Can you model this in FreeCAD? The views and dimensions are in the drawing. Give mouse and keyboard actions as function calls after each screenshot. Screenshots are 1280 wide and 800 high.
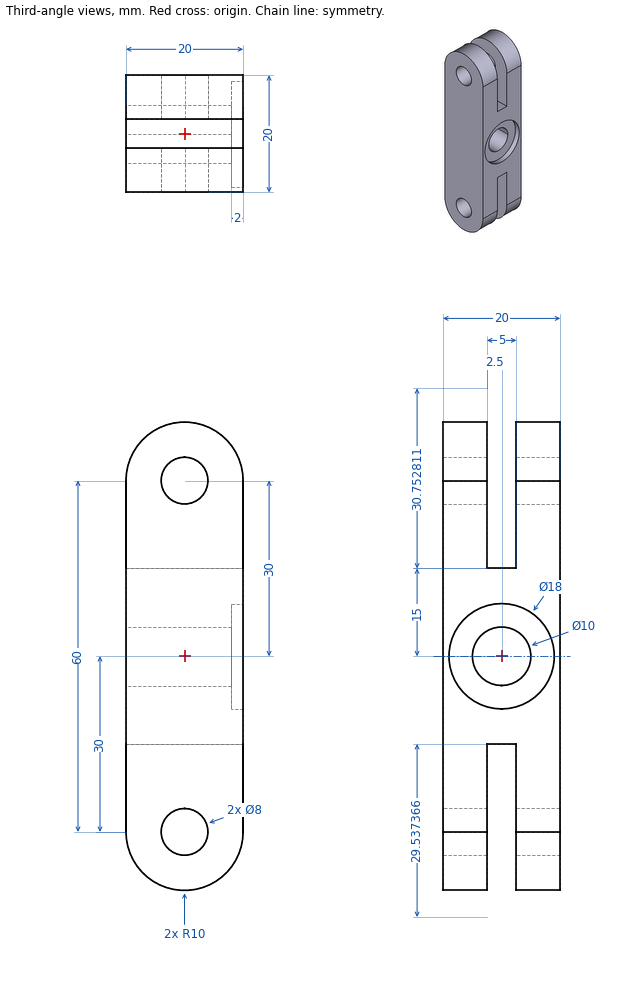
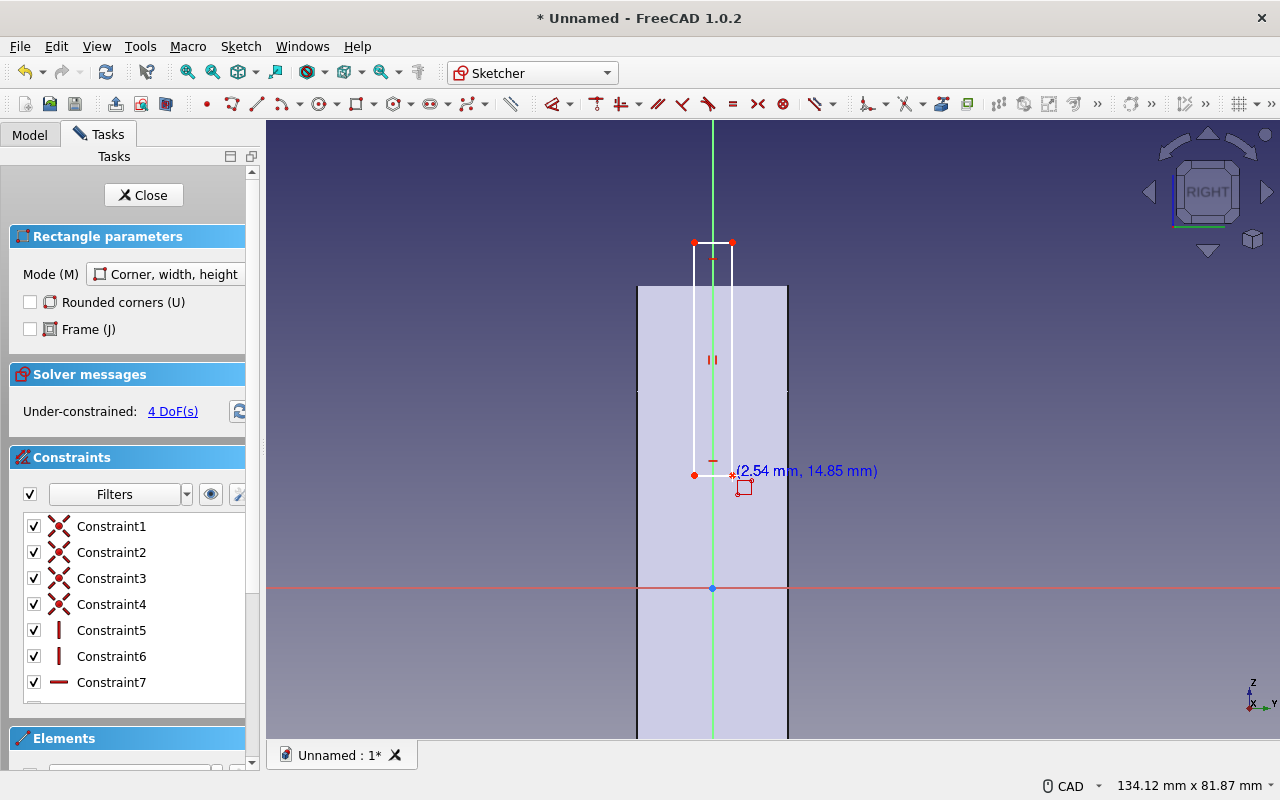
click(694, 702)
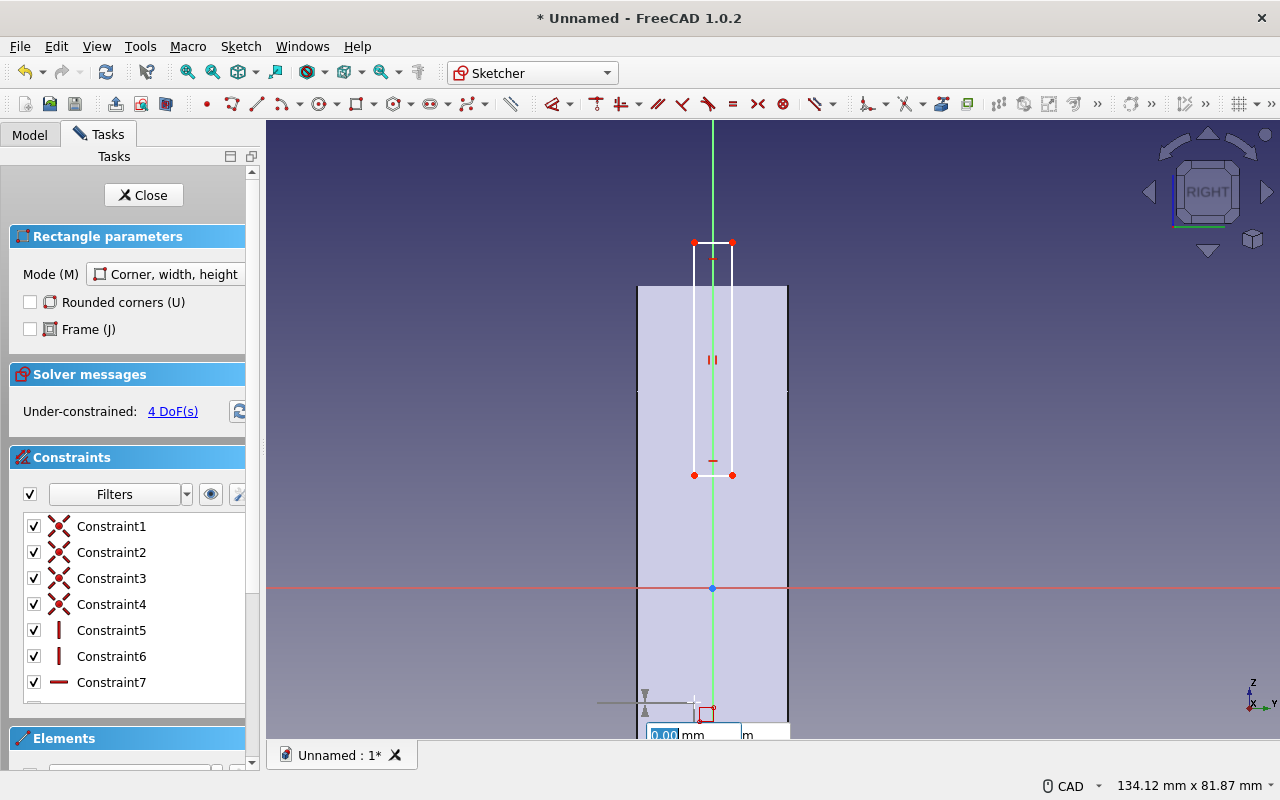
scroll(694, 242, down, 3)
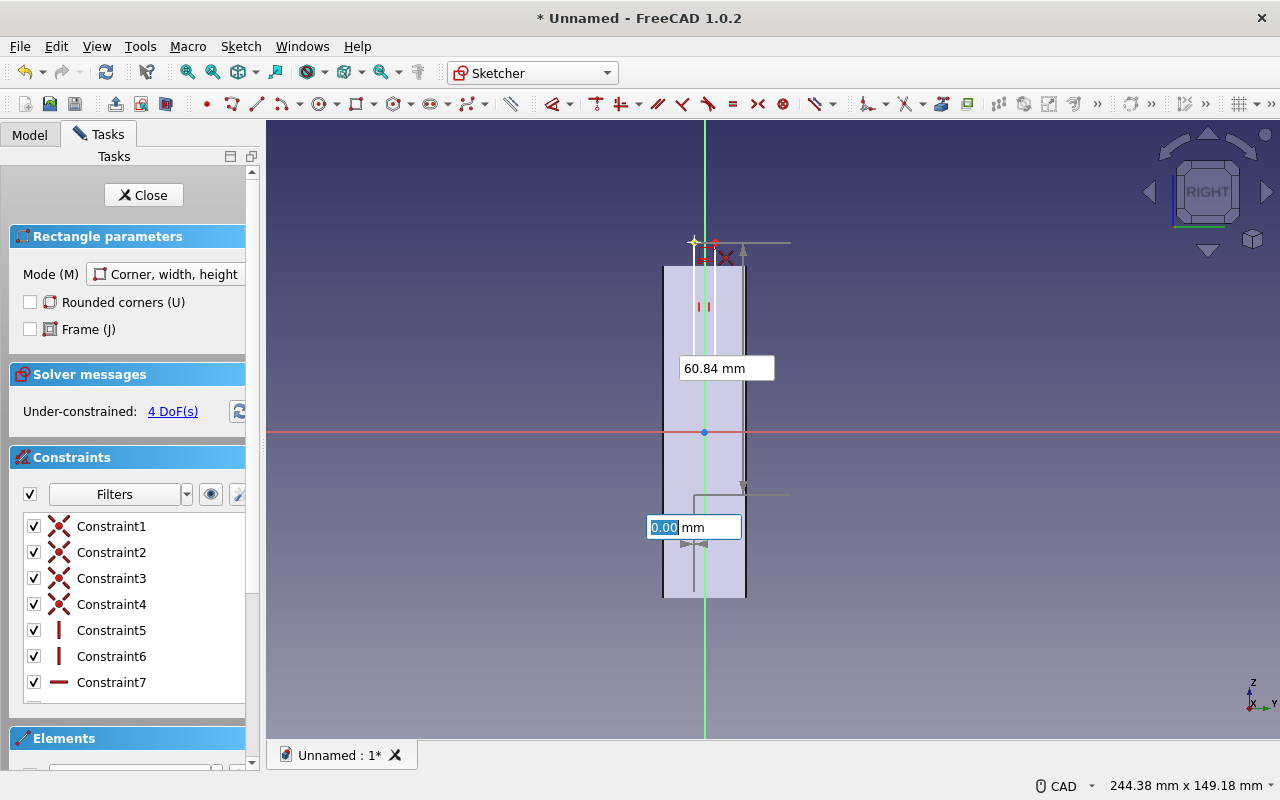
scroll(715, 617, up, 3)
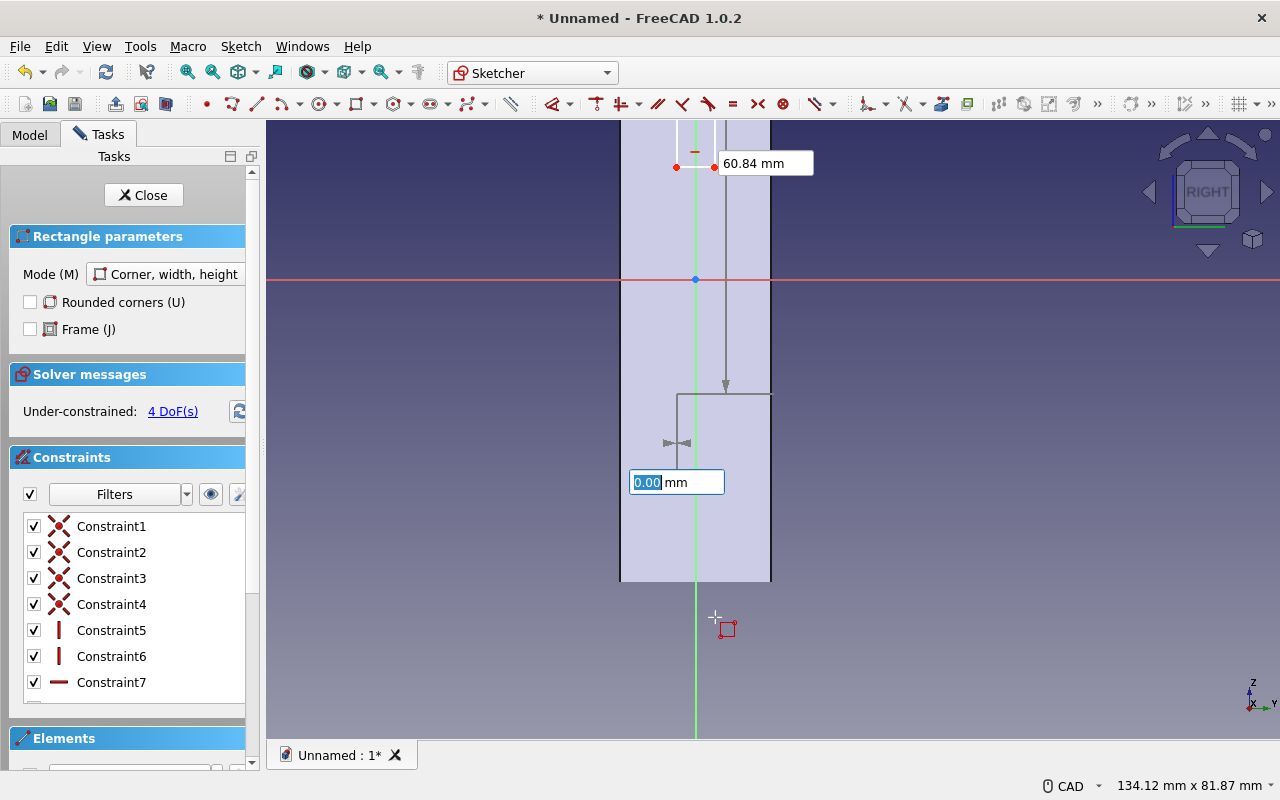
click(714, 616)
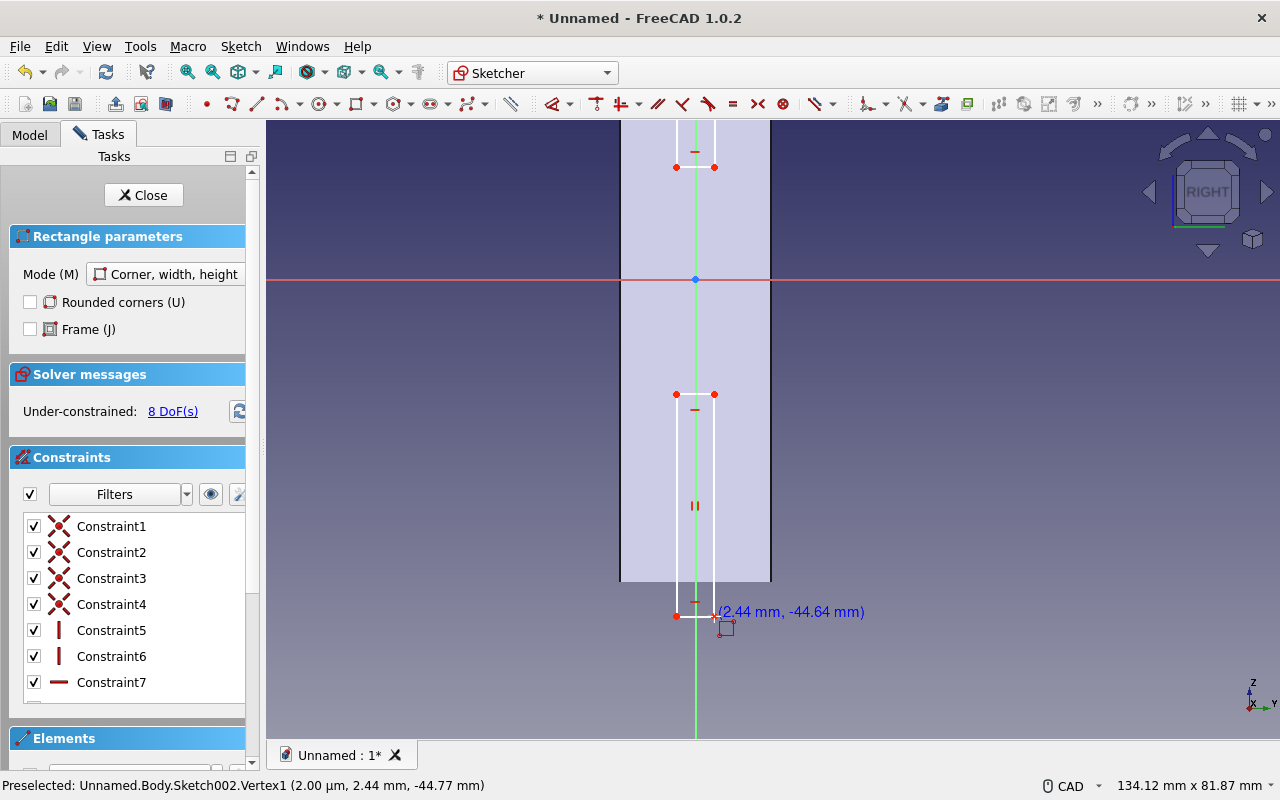
key(g)
key(c)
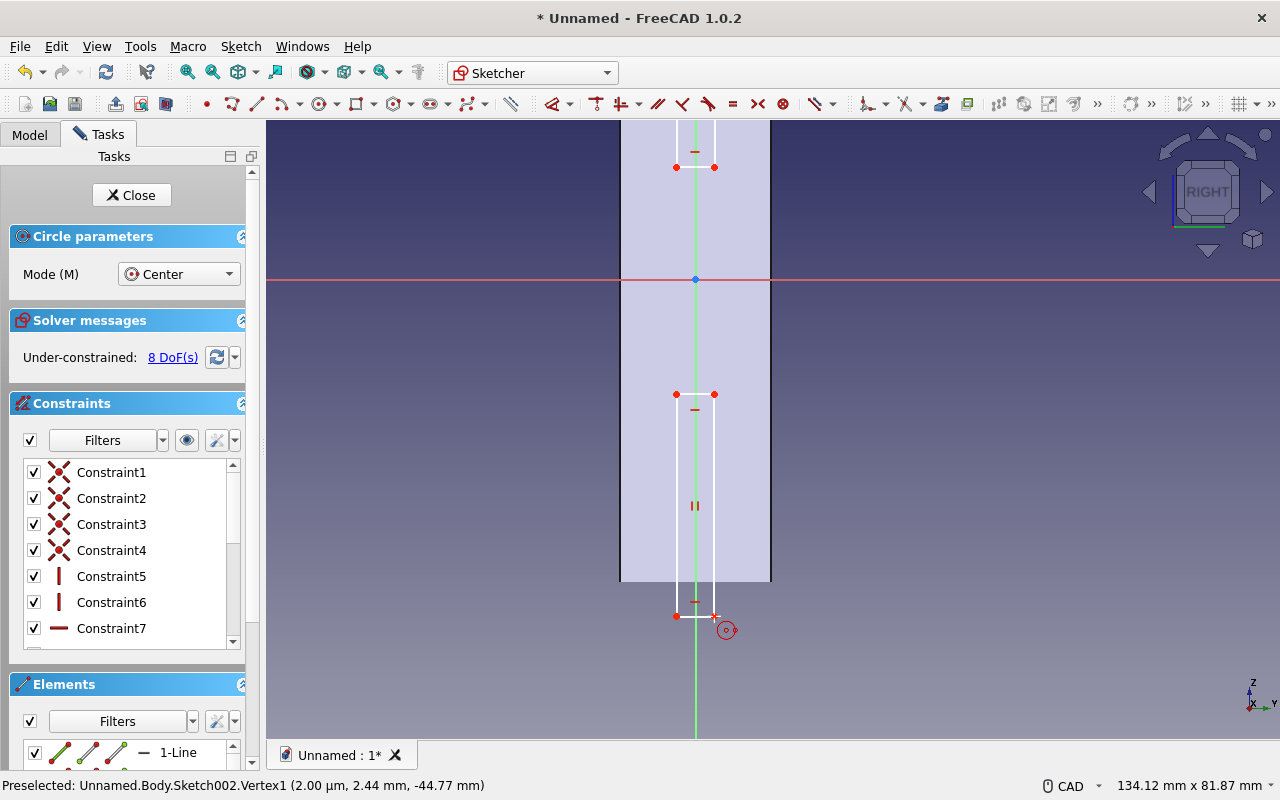
click(696, 280)
click(722, 253)
key(Escape)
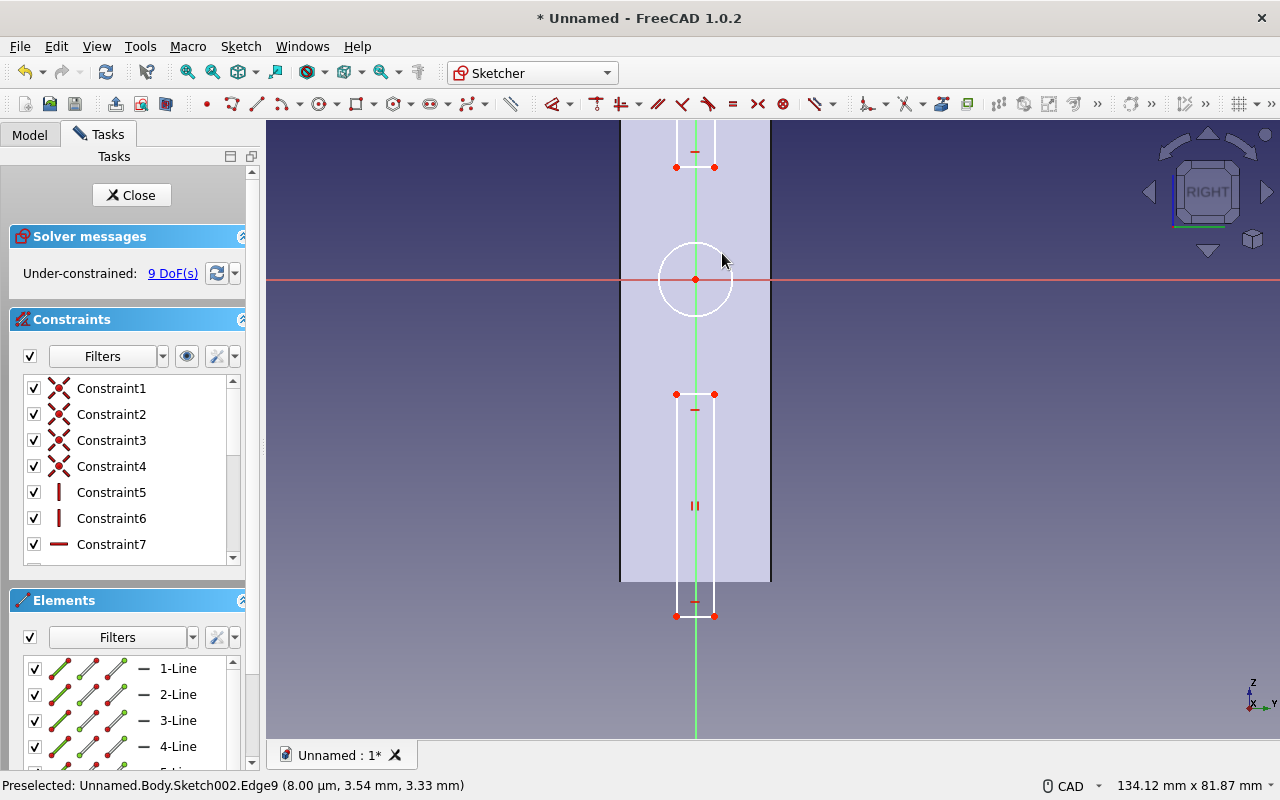
click(677, 167)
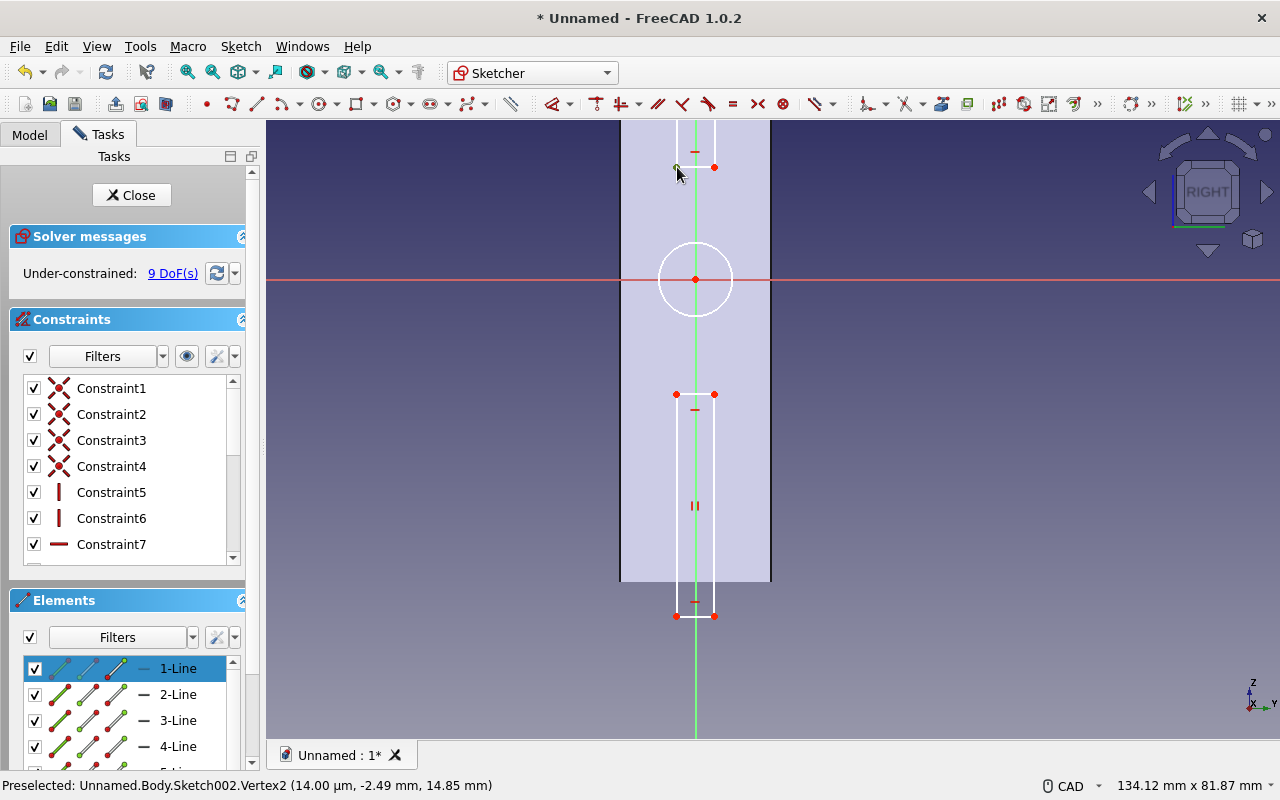
click(677, 394)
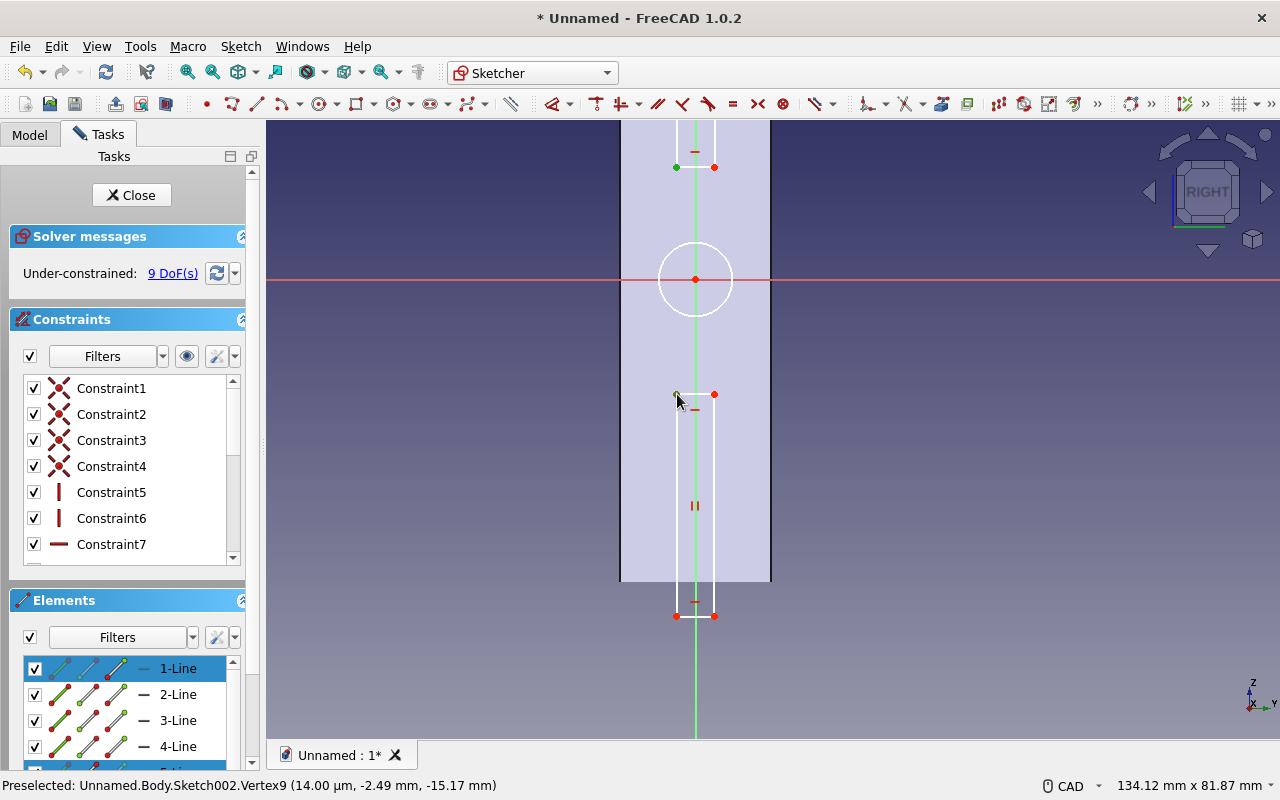
click(353, 280)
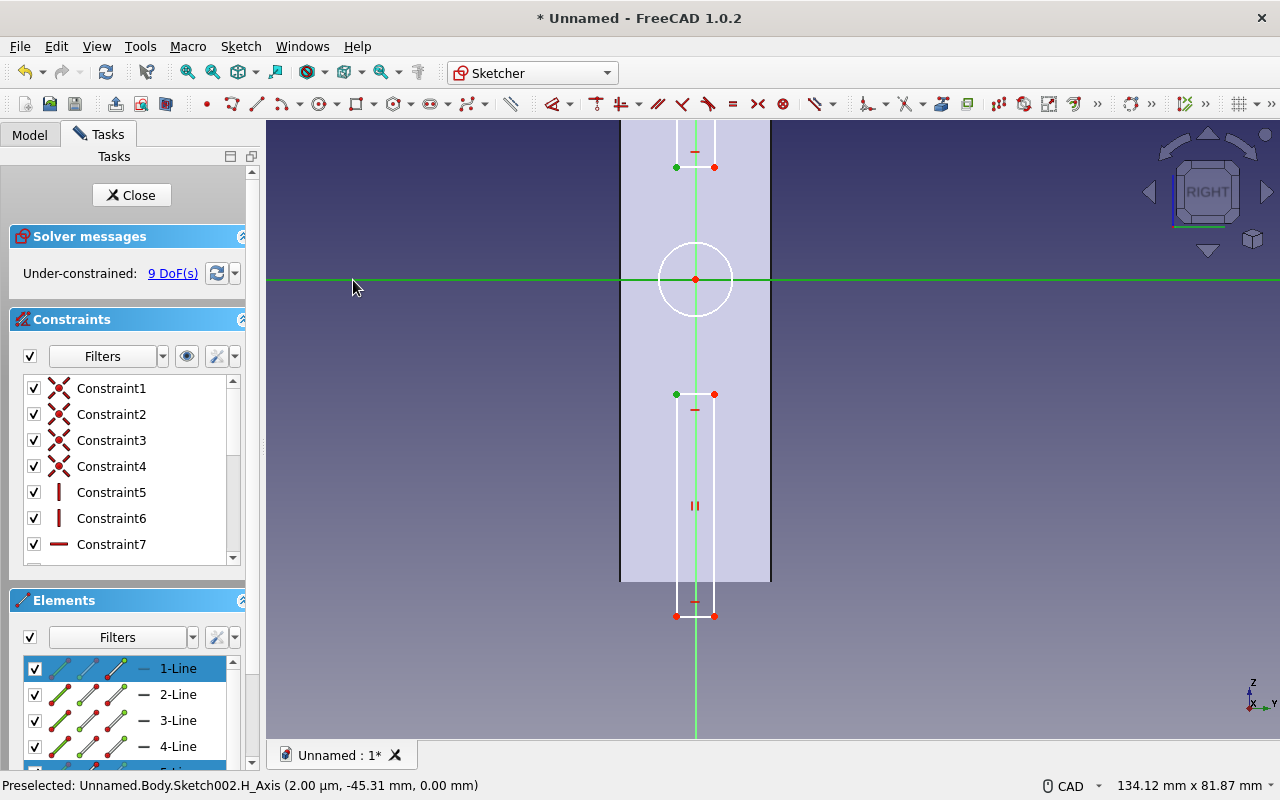
key(s)